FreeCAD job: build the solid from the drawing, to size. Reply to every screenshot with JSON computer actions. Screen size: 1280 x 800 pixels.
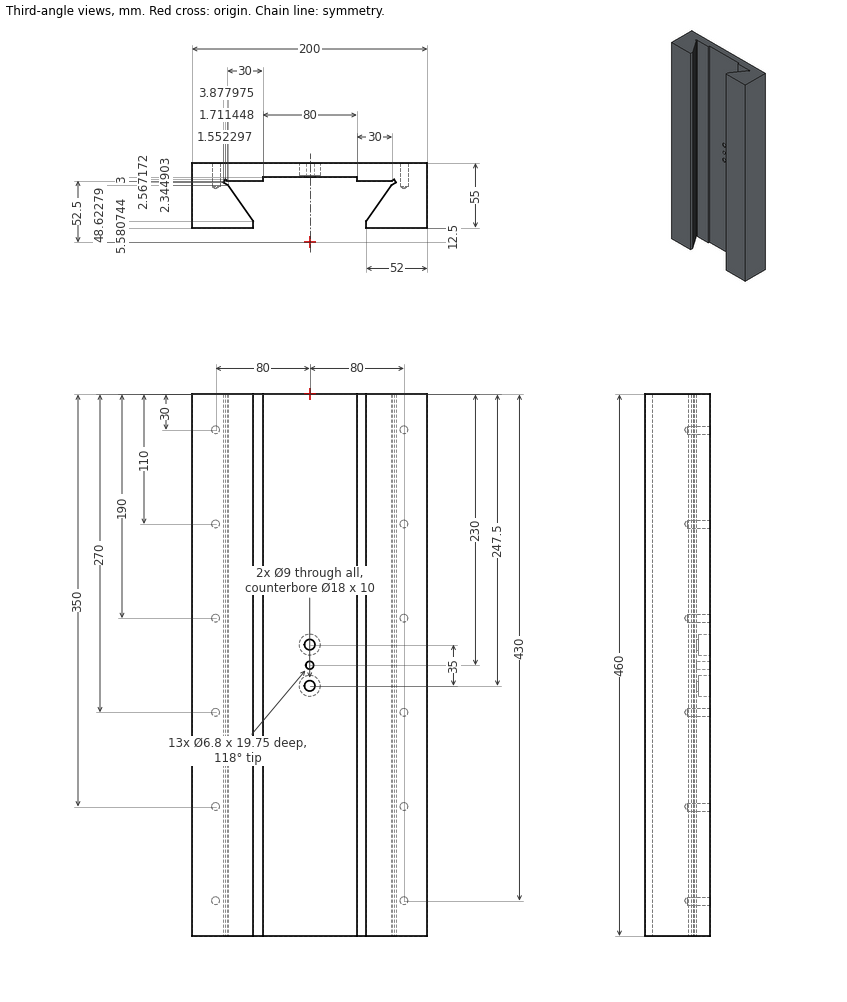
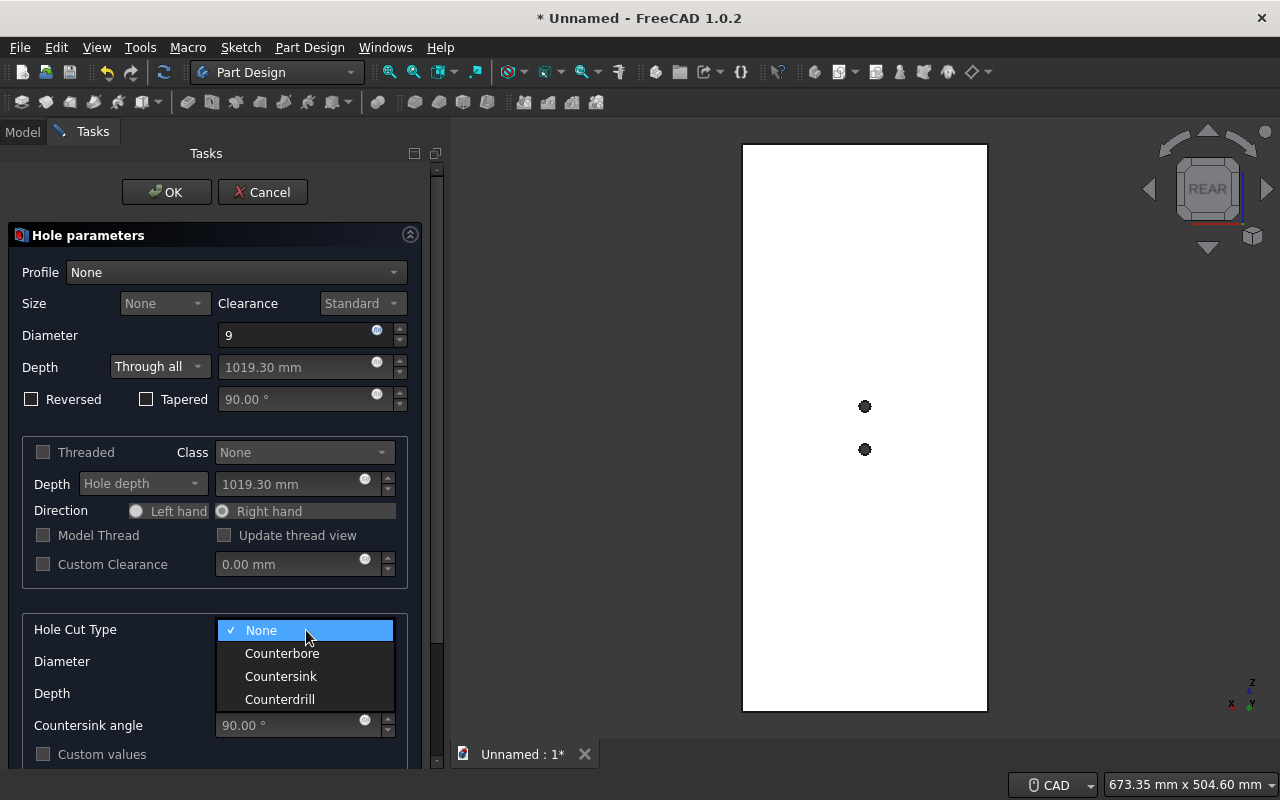
{"action": "left_click", "coordinate": [304, 654]}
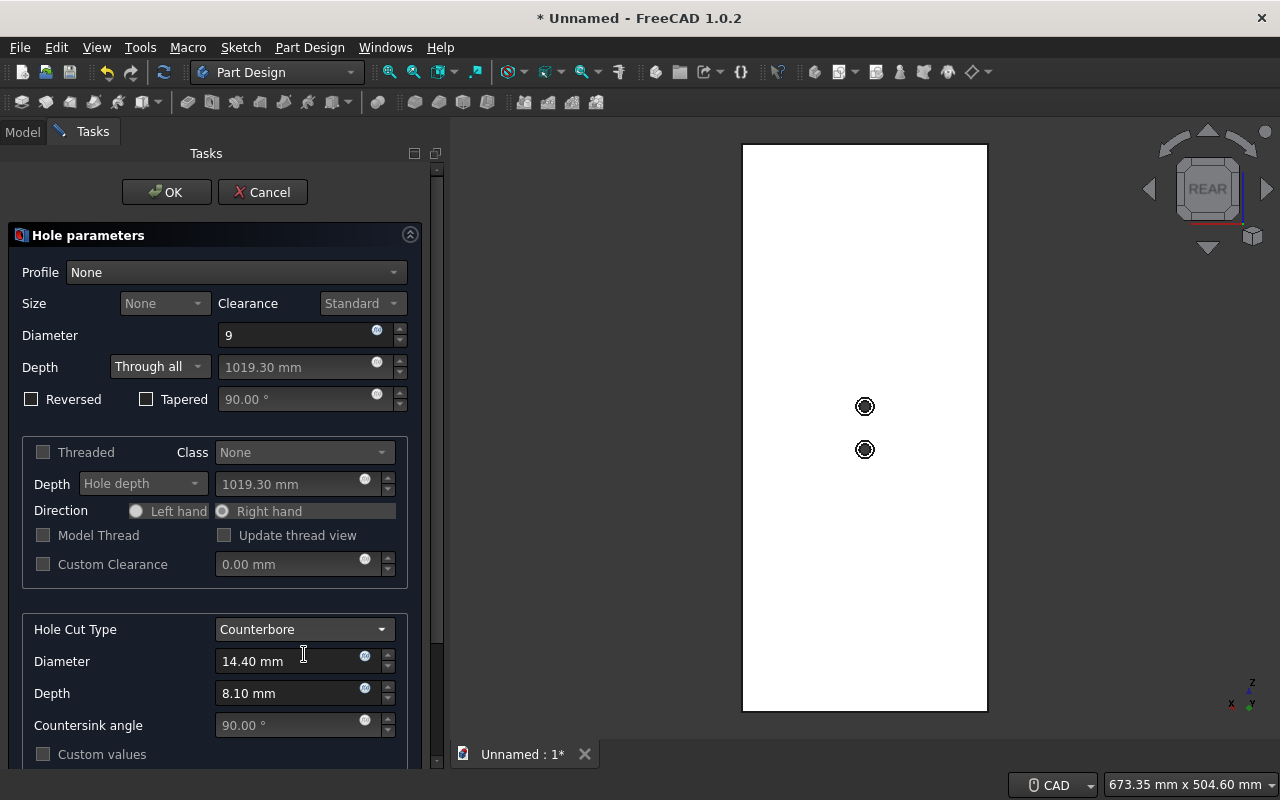
{"action": "triple_click", "coordinate": [298, 661]}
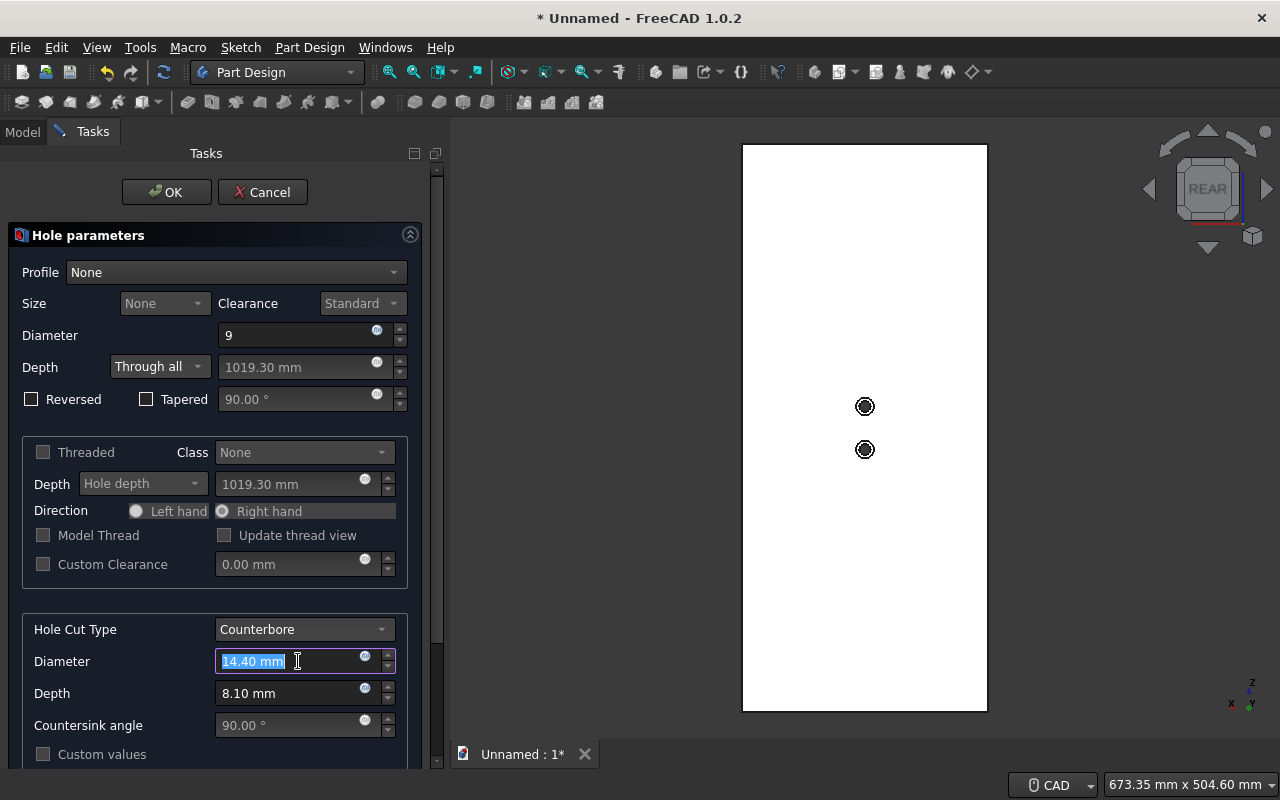
{"action": "type", "text": "18"}
{"action": "key", "text": "Tab"}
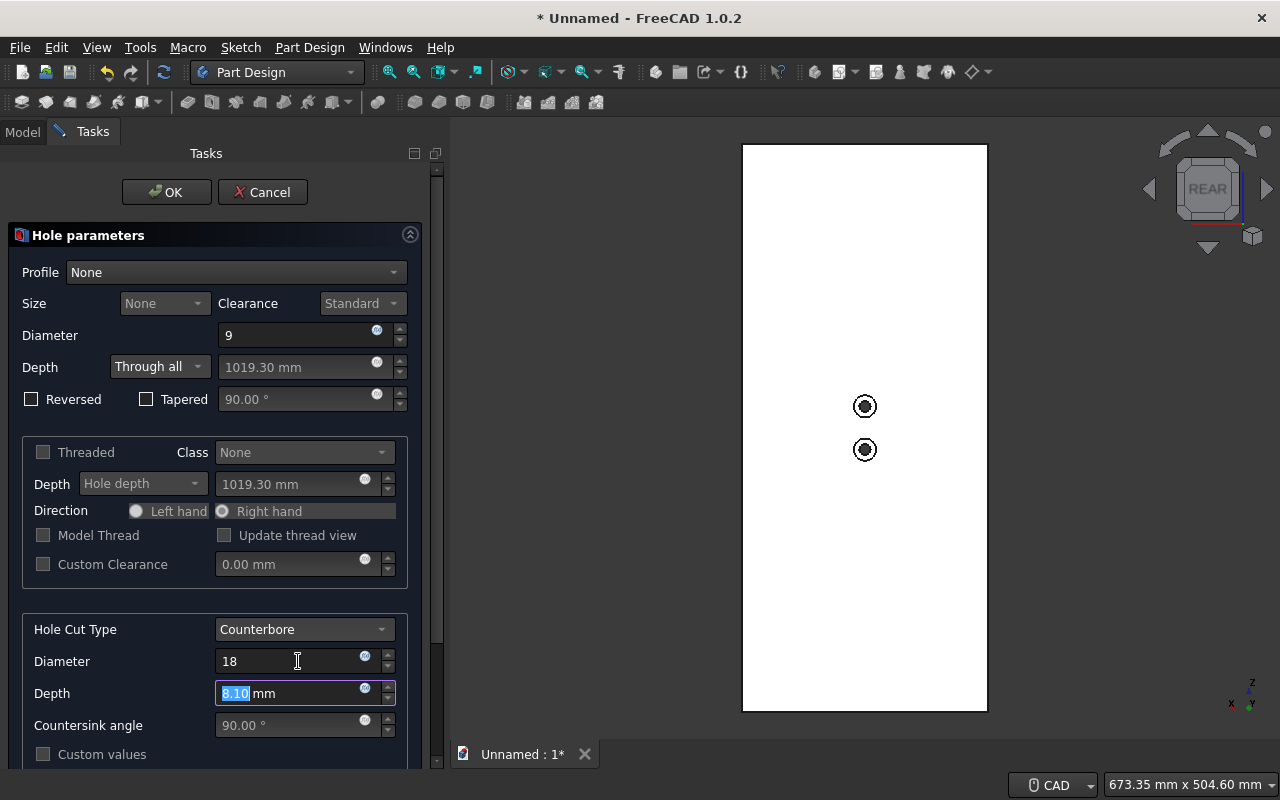
{"action": "type", "text": "10"}
{"action": "key", "text": "Tab"}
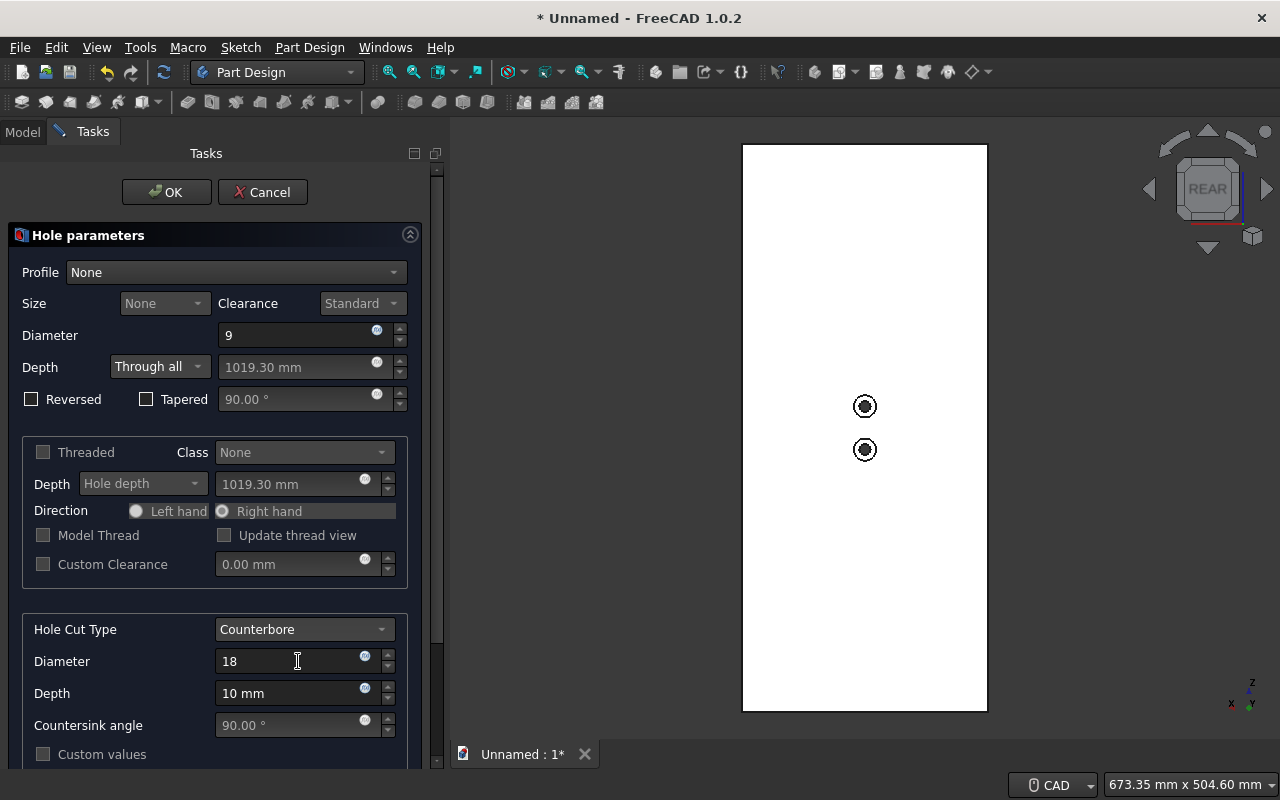
{"action": "left_click", "coordinate": [167, 192]}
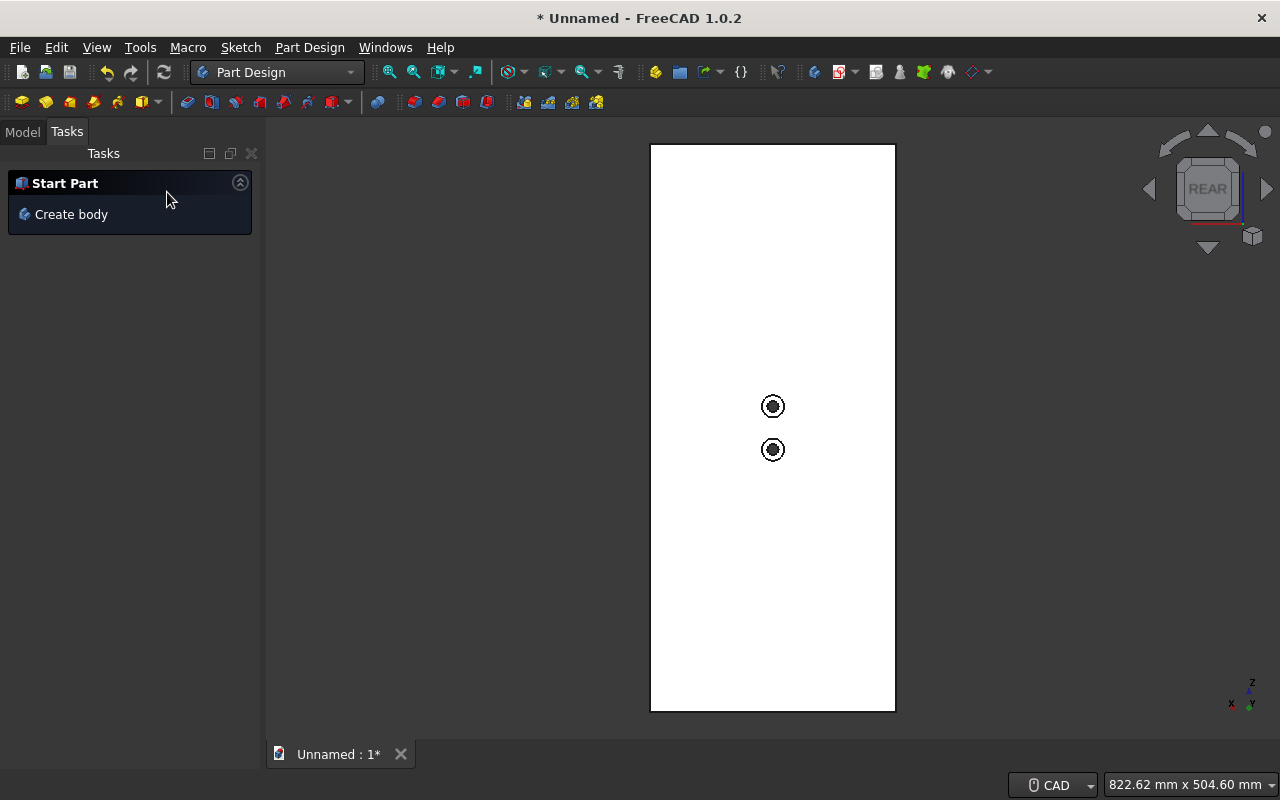
{"action": "left_click", "coordinate": [773, 265]}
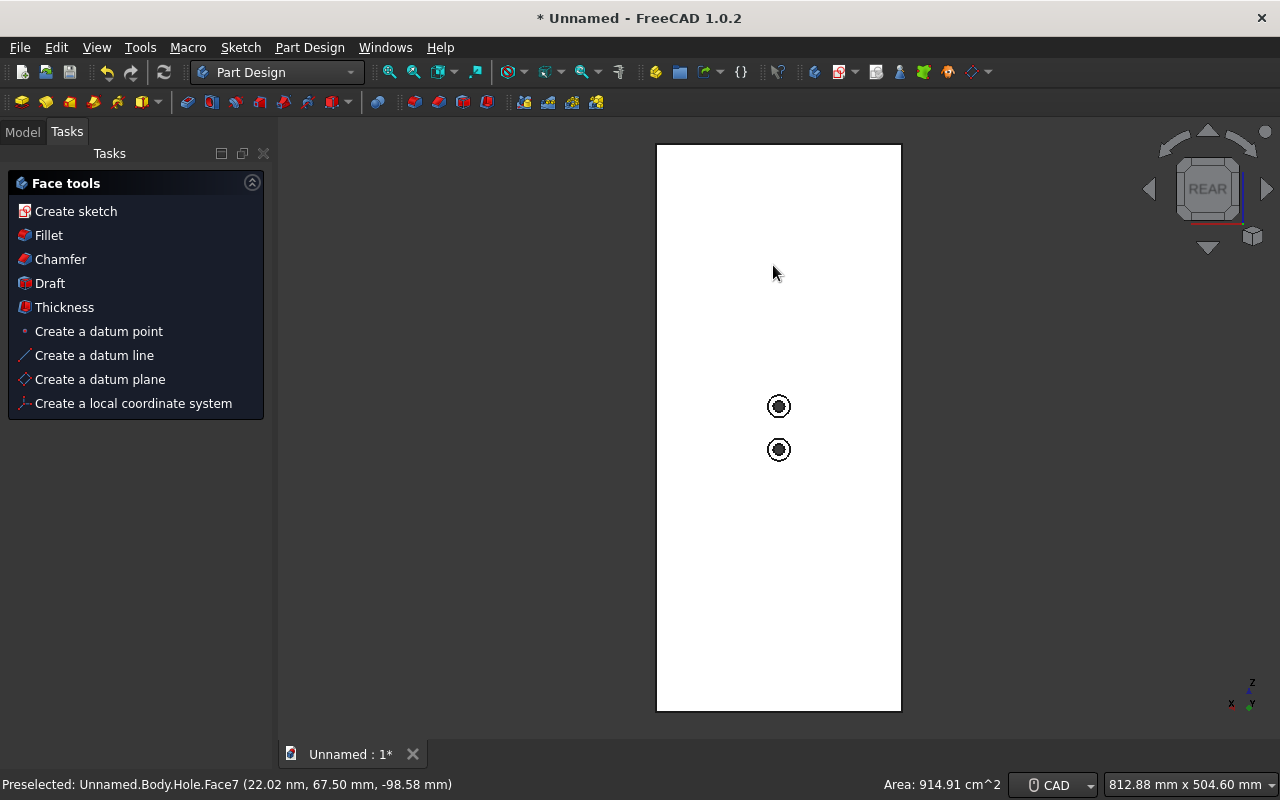
{"action": "left_click", "coordinate": [840, 72]}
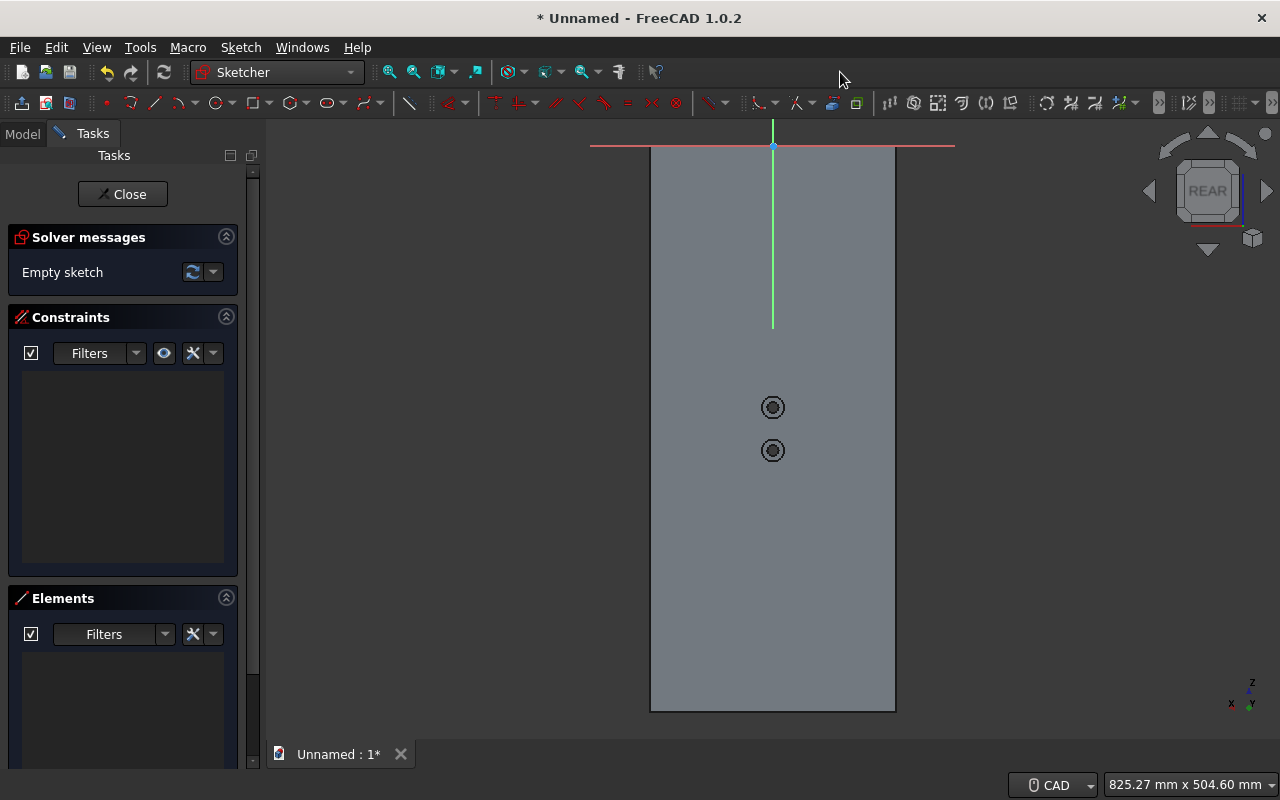
{"action": "scroll", "coordinate": [395, 503], "scroll_direction": "down", "scroll_amount": 1}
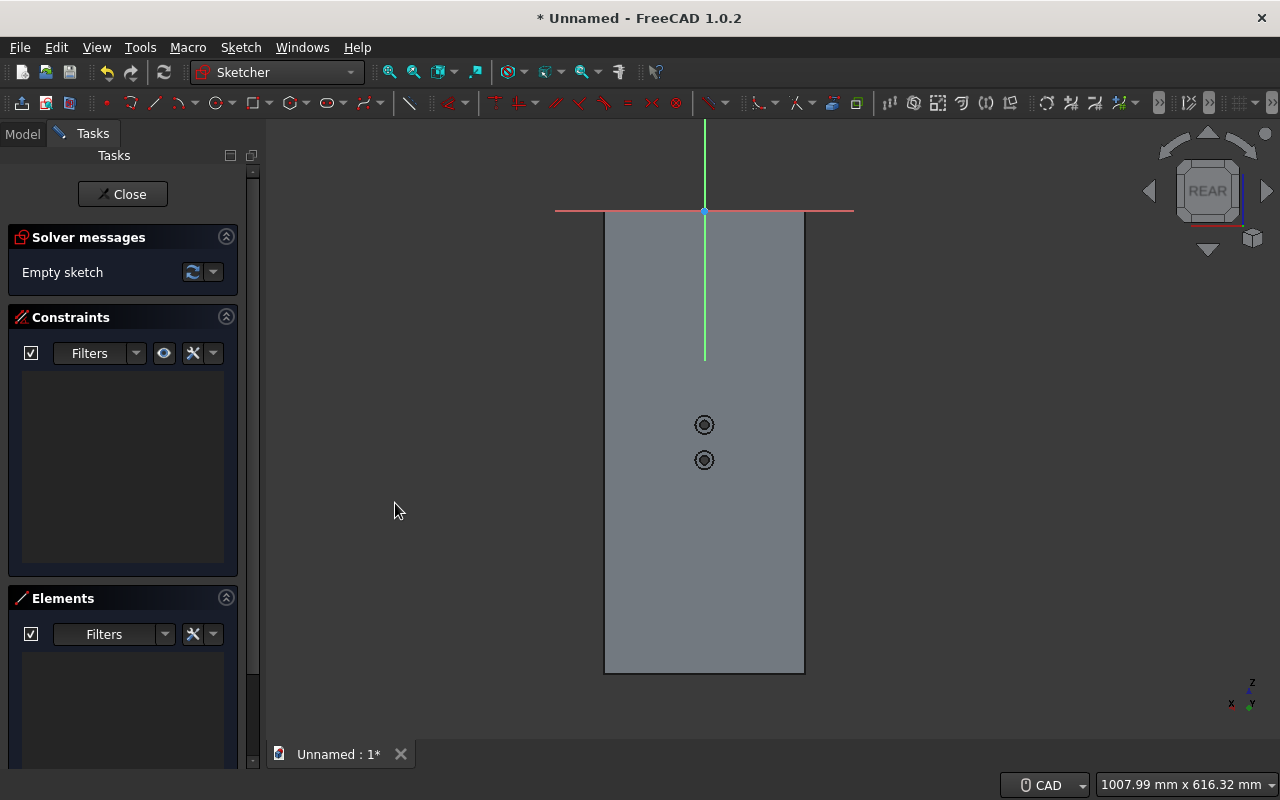
{"action": "left_click", "coordinate": [216, 104]}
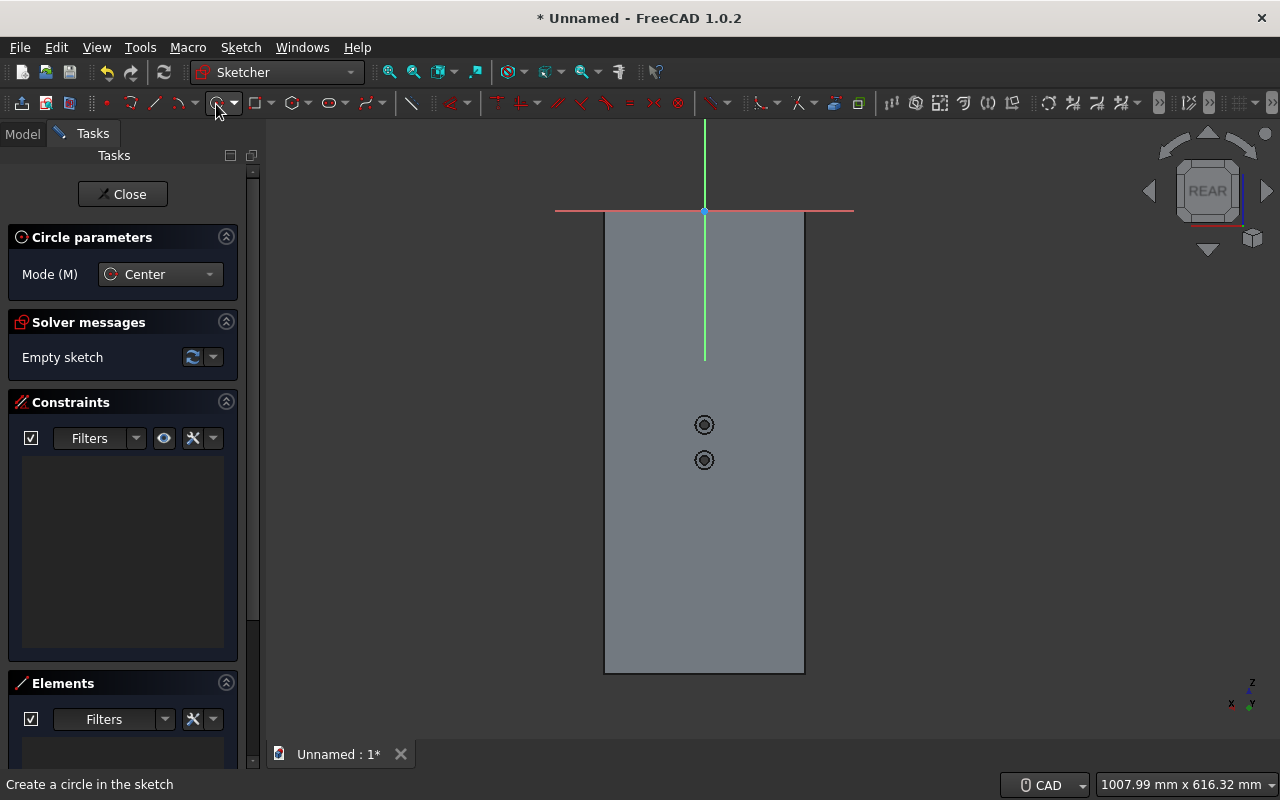
{"action": "scroll", "coordinate": [705, 443], "scroll_direction": "up", "scroll_amount": 10}